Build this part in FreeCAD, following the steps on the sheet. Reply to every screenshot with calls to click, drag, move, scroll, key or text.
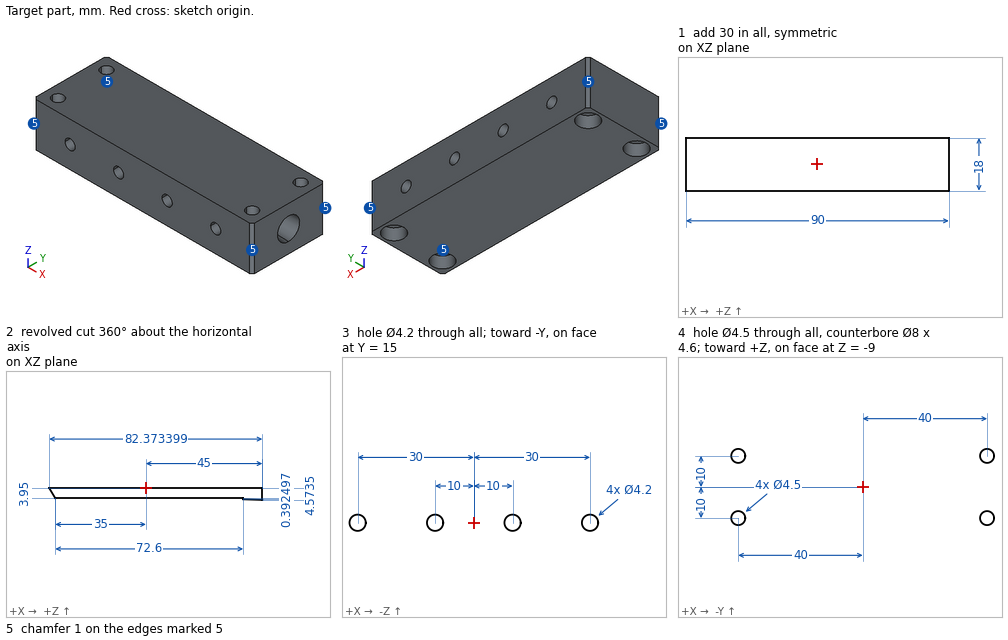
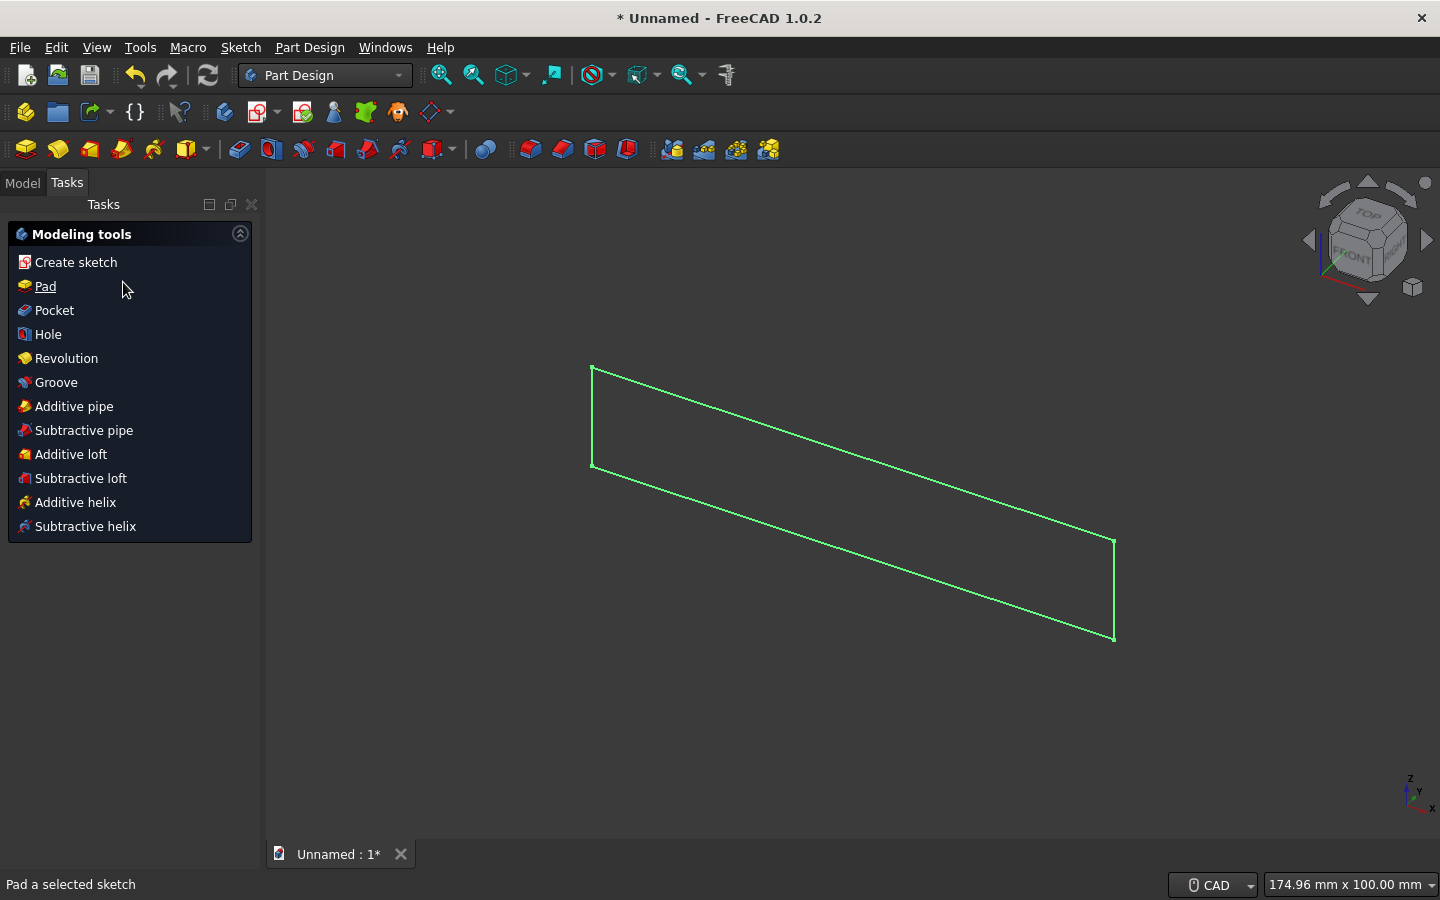
click(26, 150)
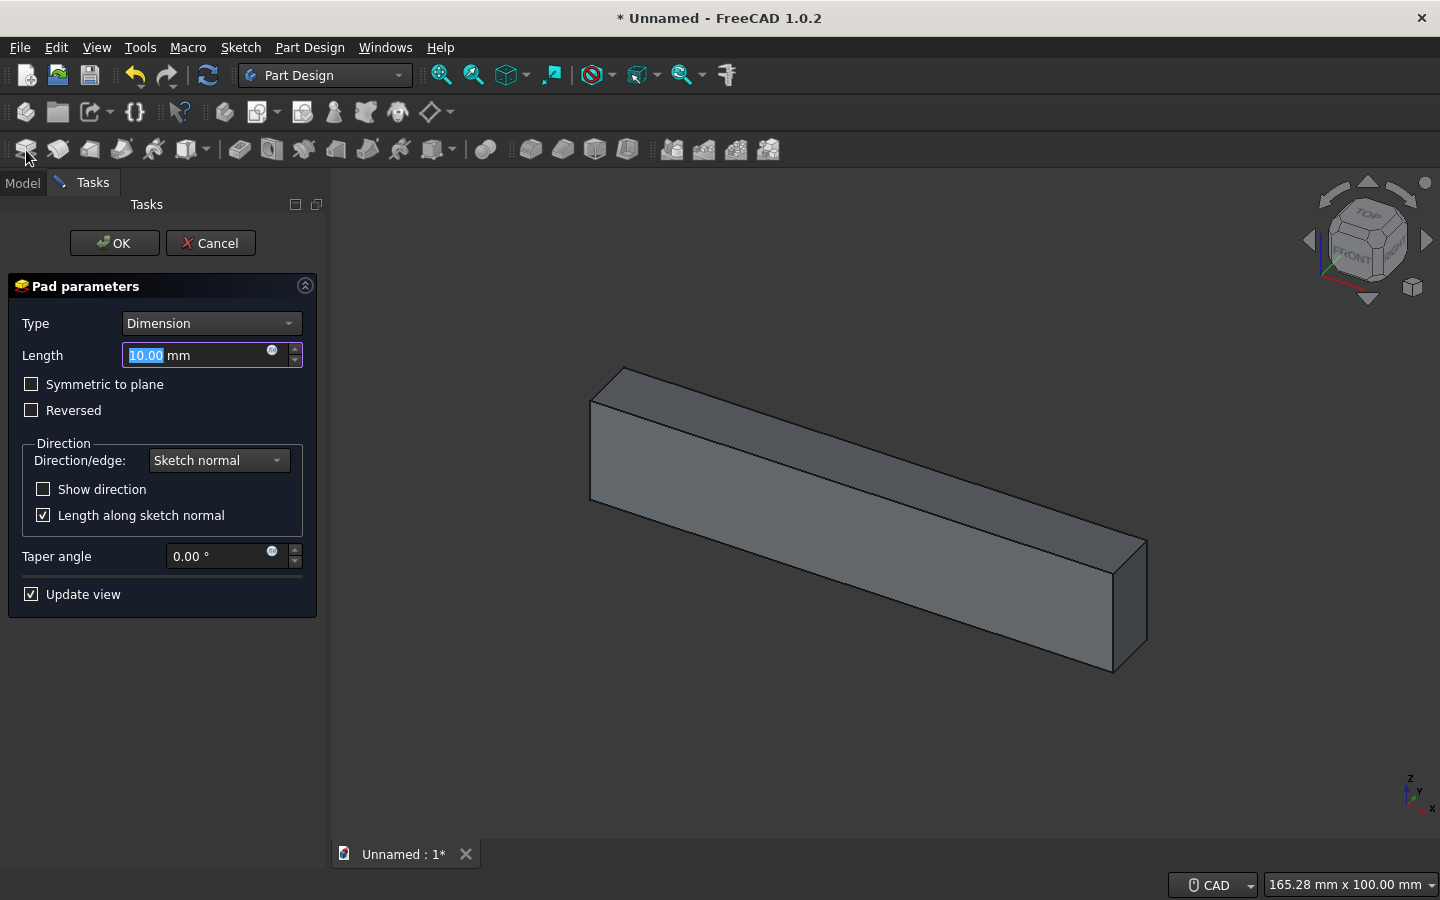
text(30)
key(Tab)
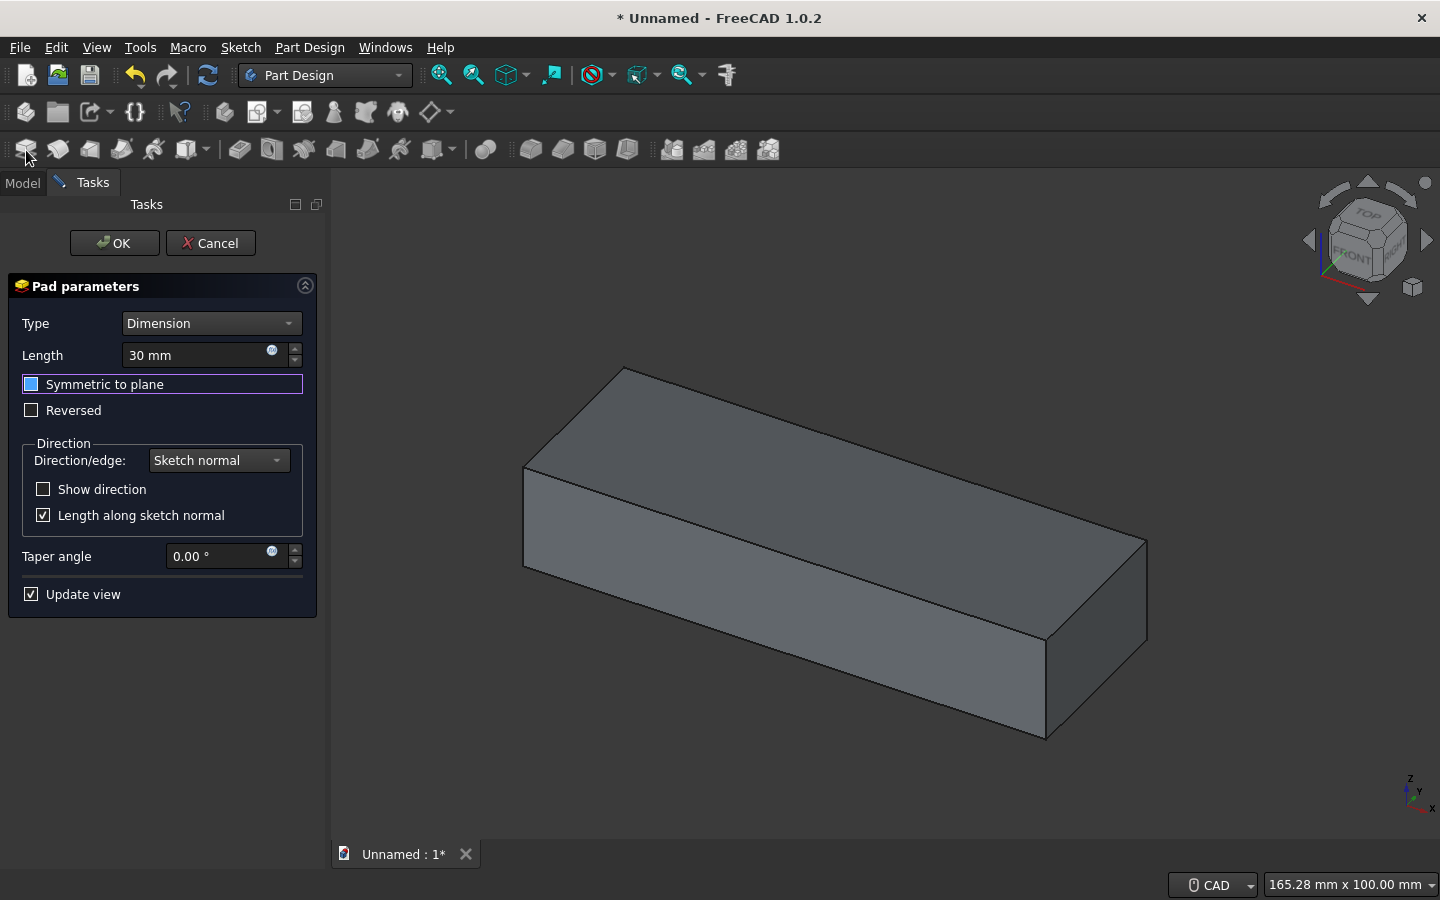
click(30, 384)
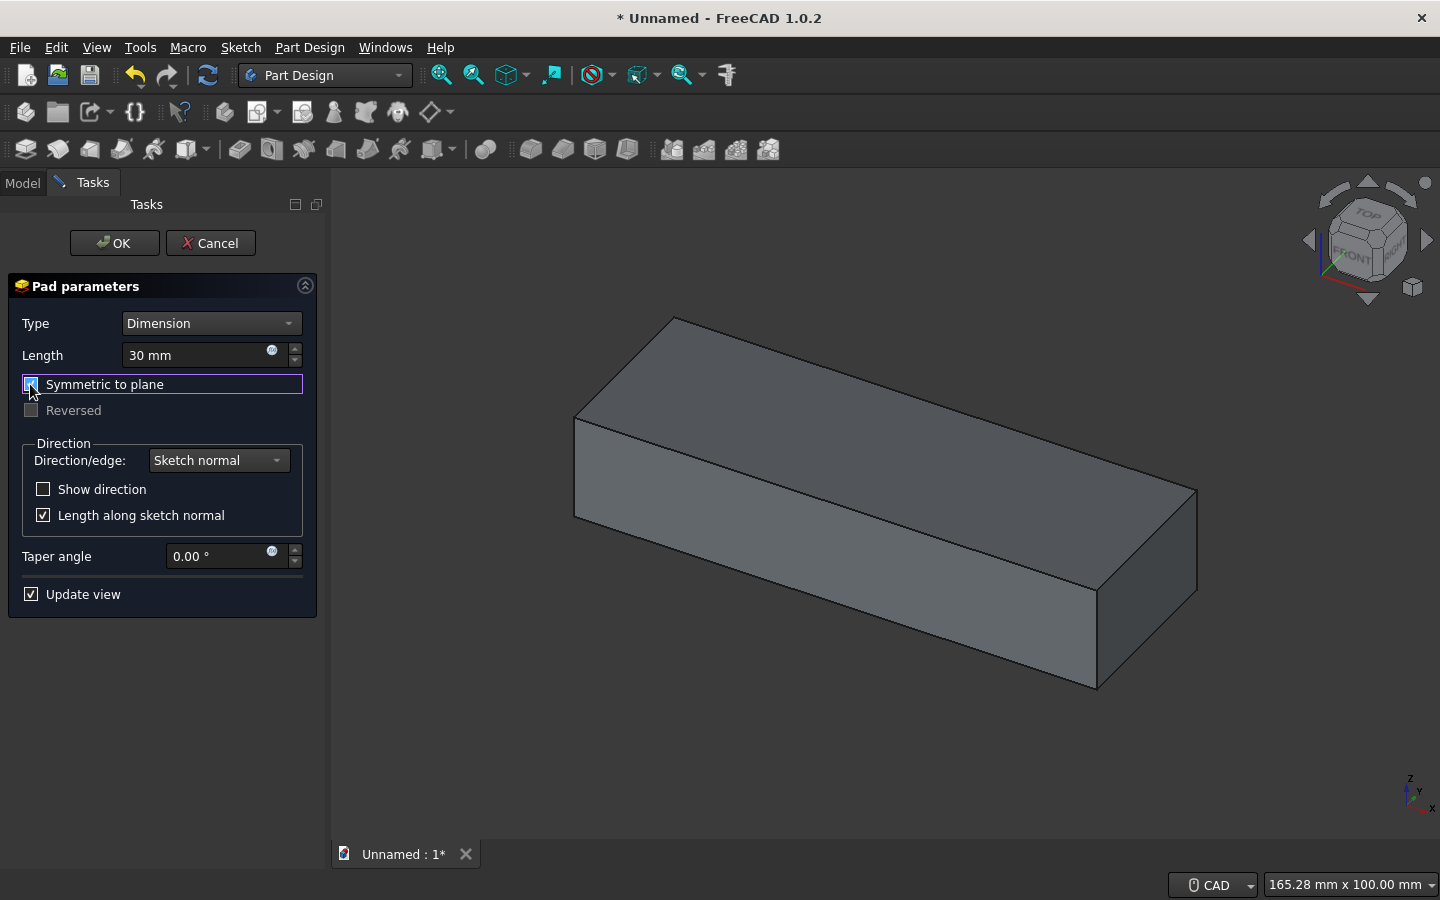
click(115, 243)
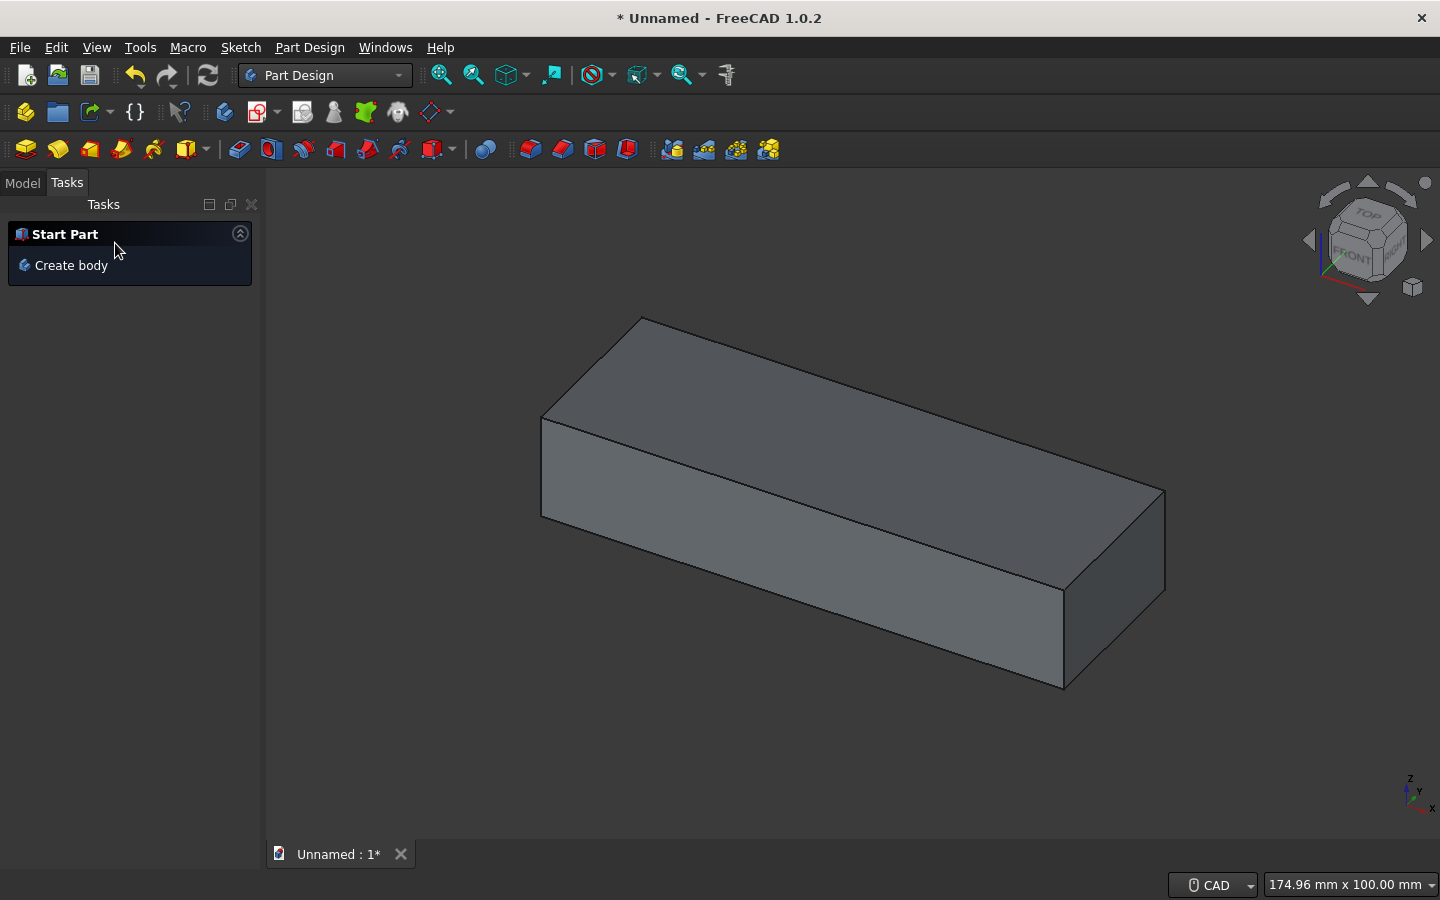
click(258, 112)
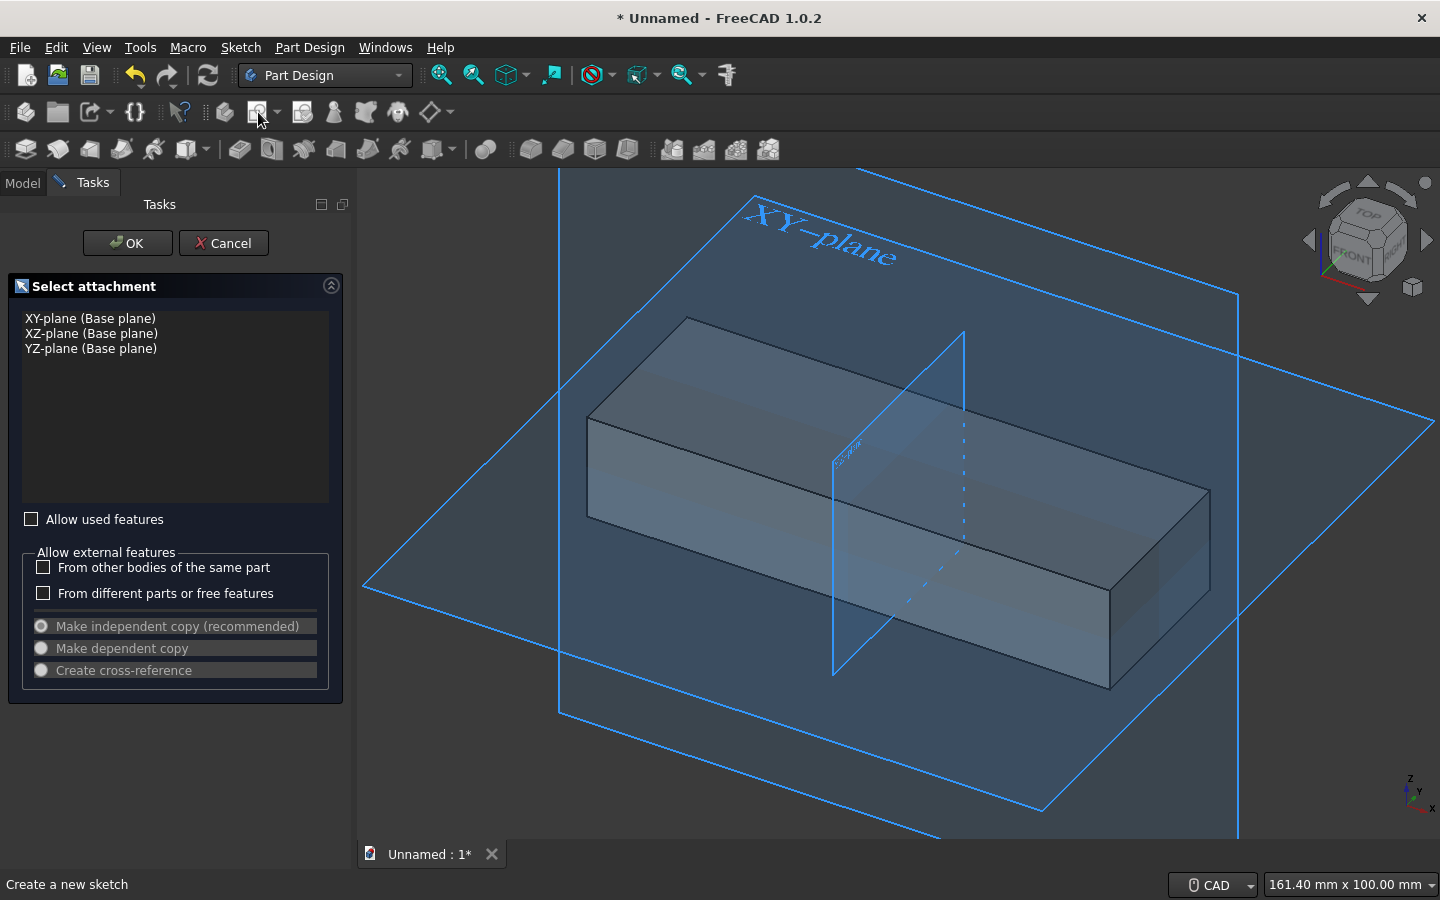
click(82, 334)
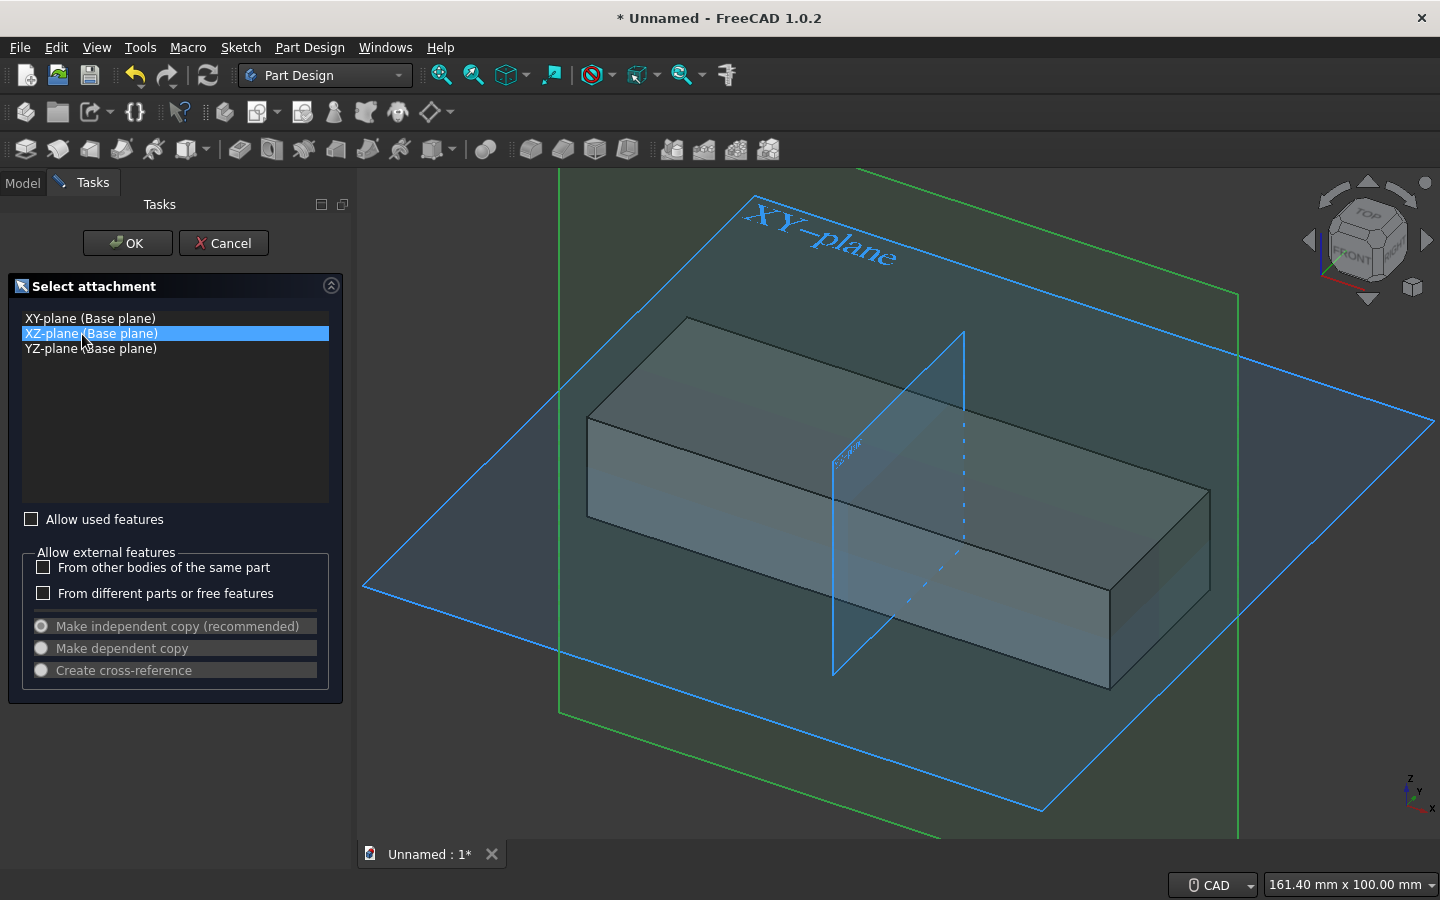
click(128, 243)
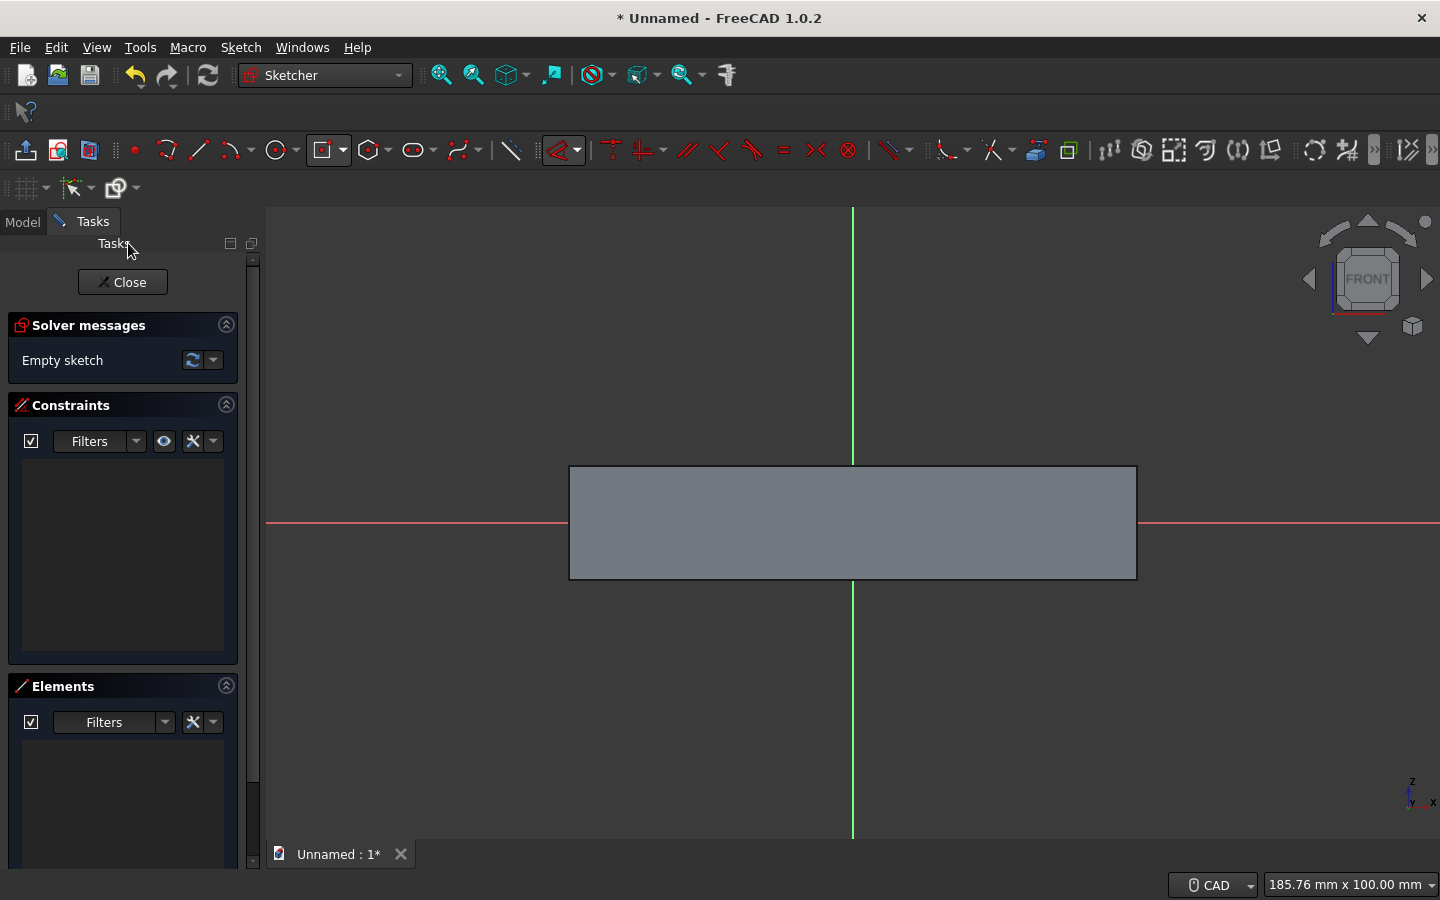
click(90, 150)